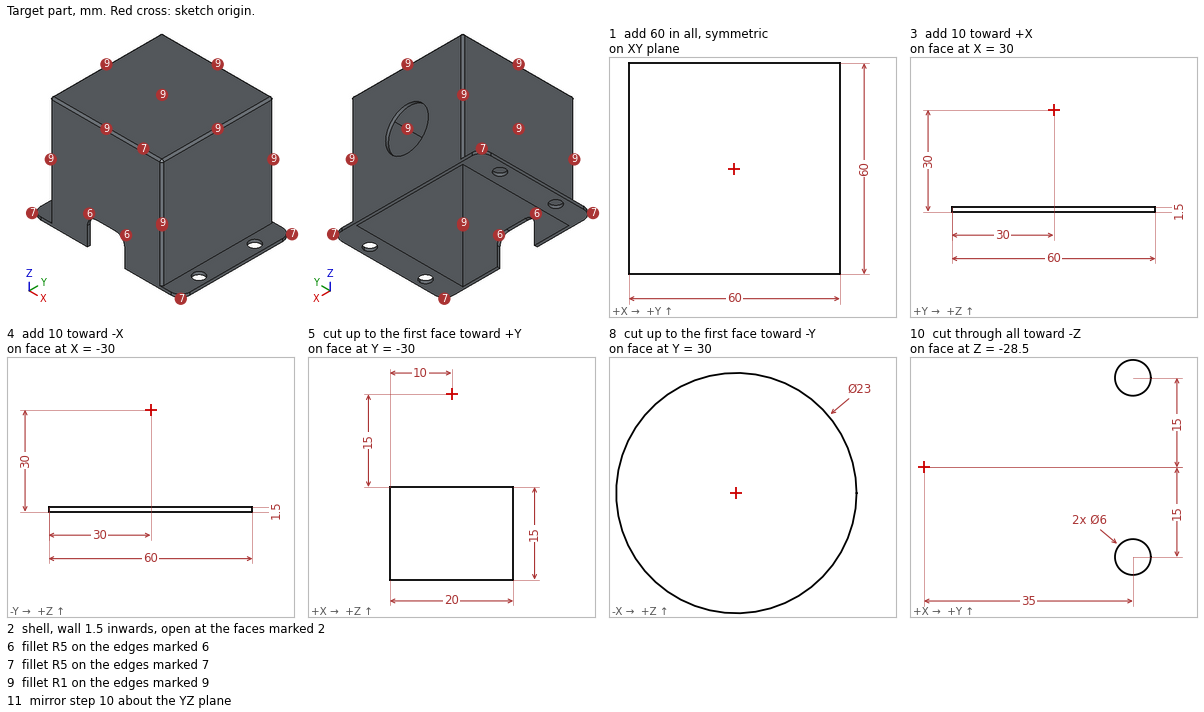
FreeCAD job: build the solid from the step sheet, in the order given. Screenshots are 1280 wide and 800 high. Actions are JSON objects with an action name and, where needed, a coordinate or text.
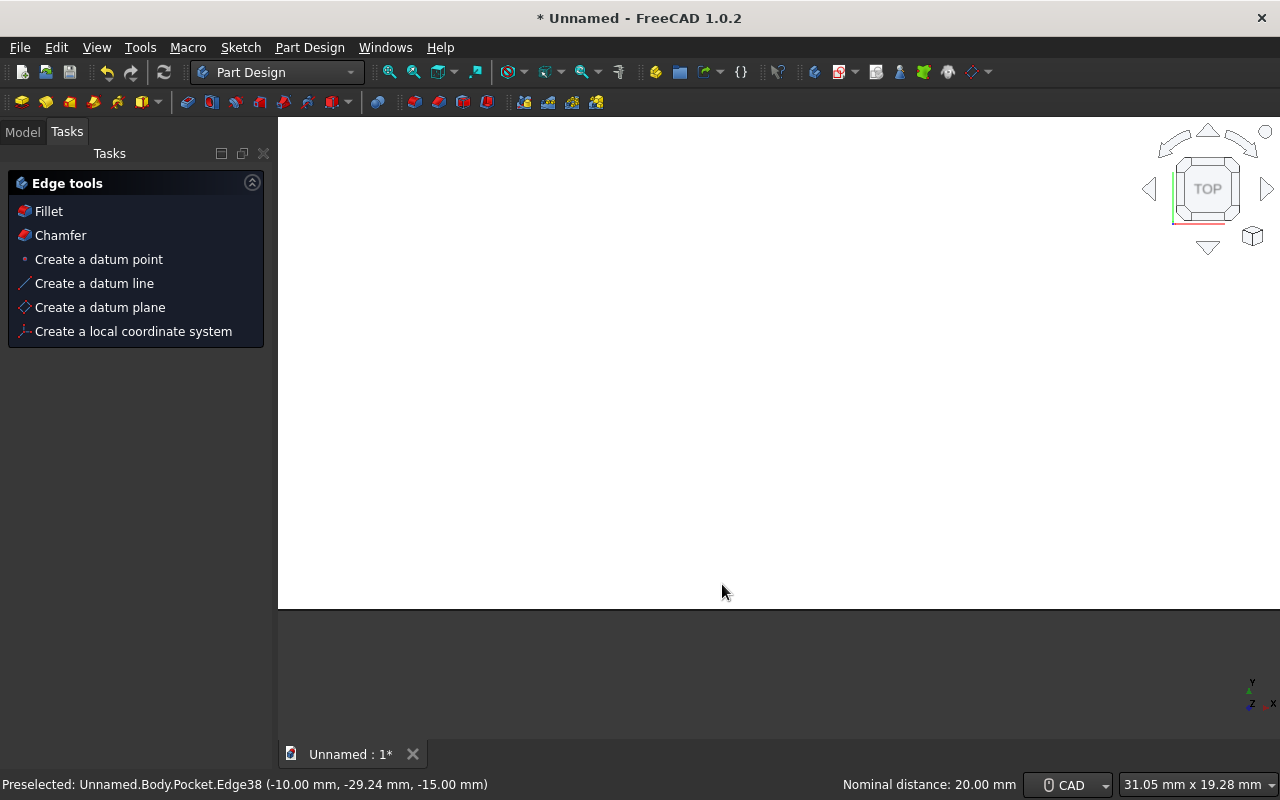
{"action": "left_click", "coordinate": [416, 102]}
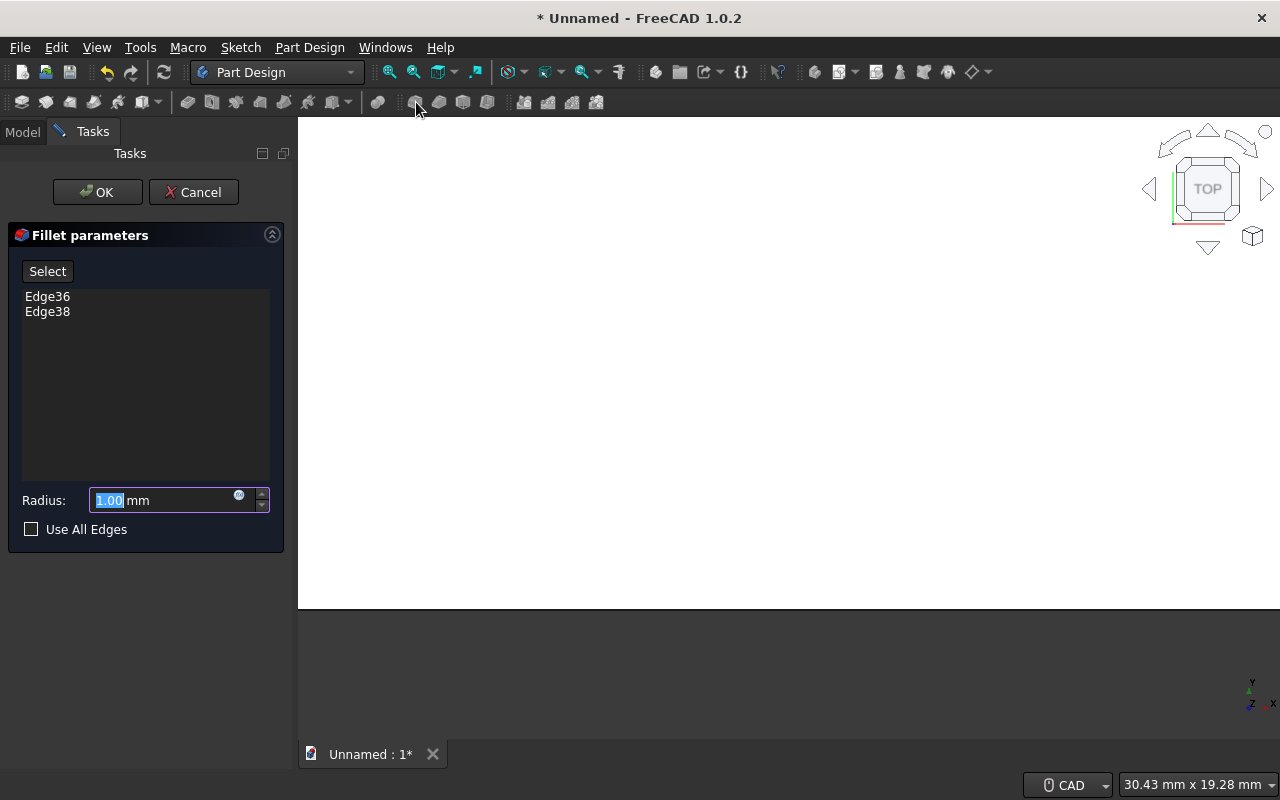
{"action": "type", "text": "5"}
{"action": "key", "text": "Tab"}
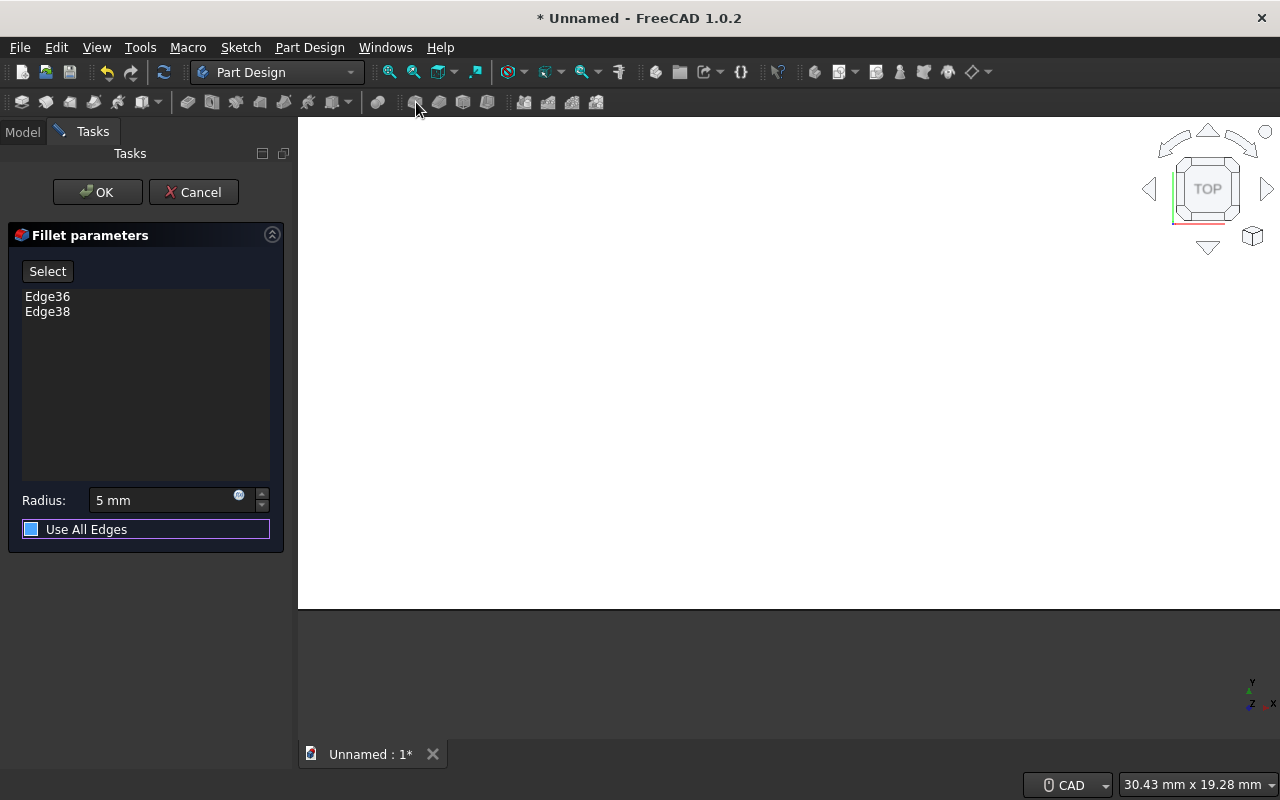
{"action": "left_click", "coordinate": [98, 192]}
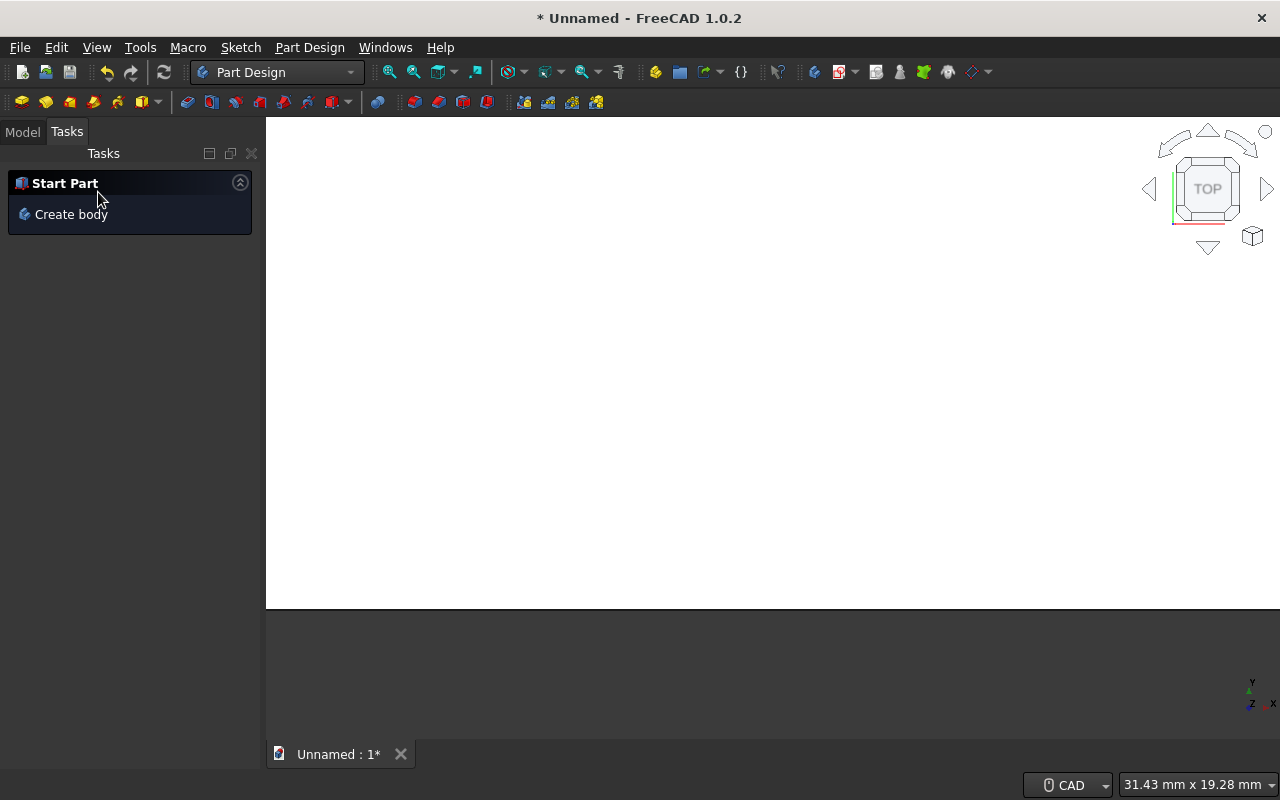
{"action": "key", "text": "v f"}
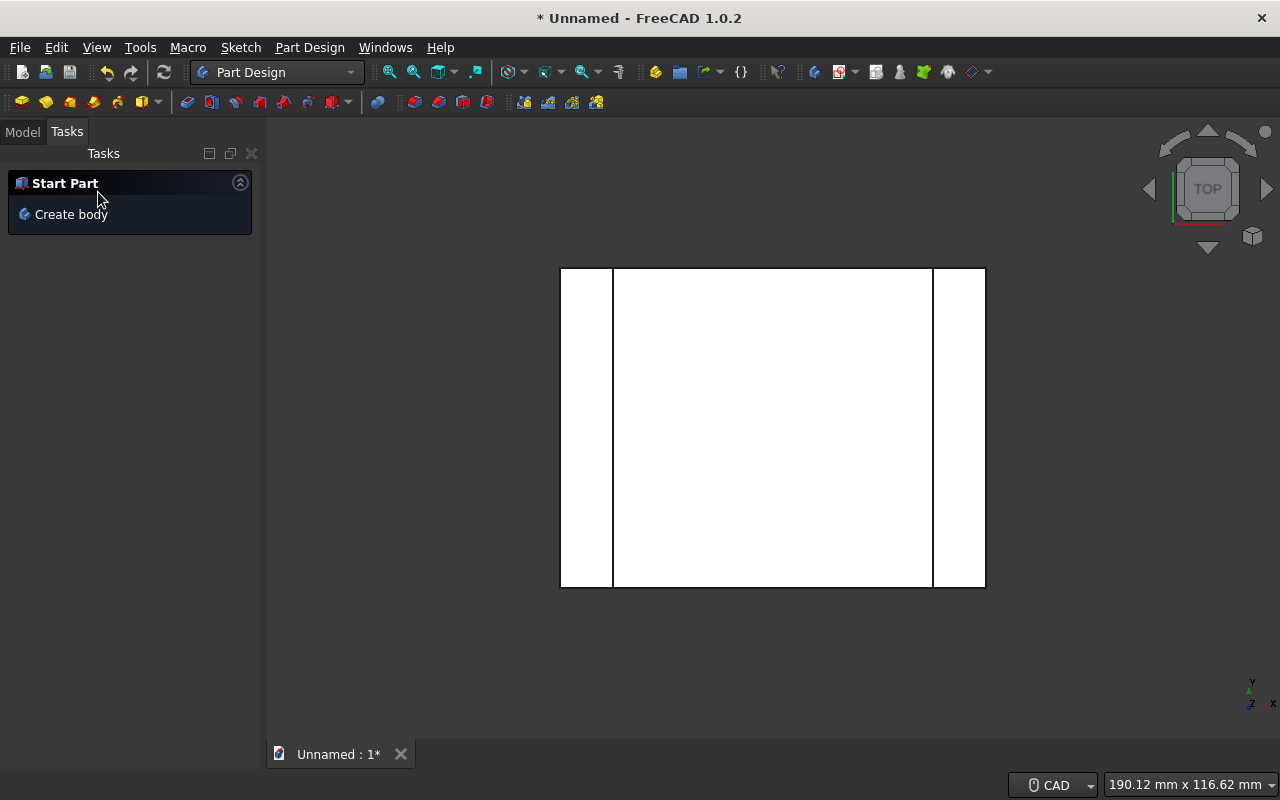
{"action": "scroll", "coordinate": [986, 267], "scroll_direction": "up", "scroll_amount": 9}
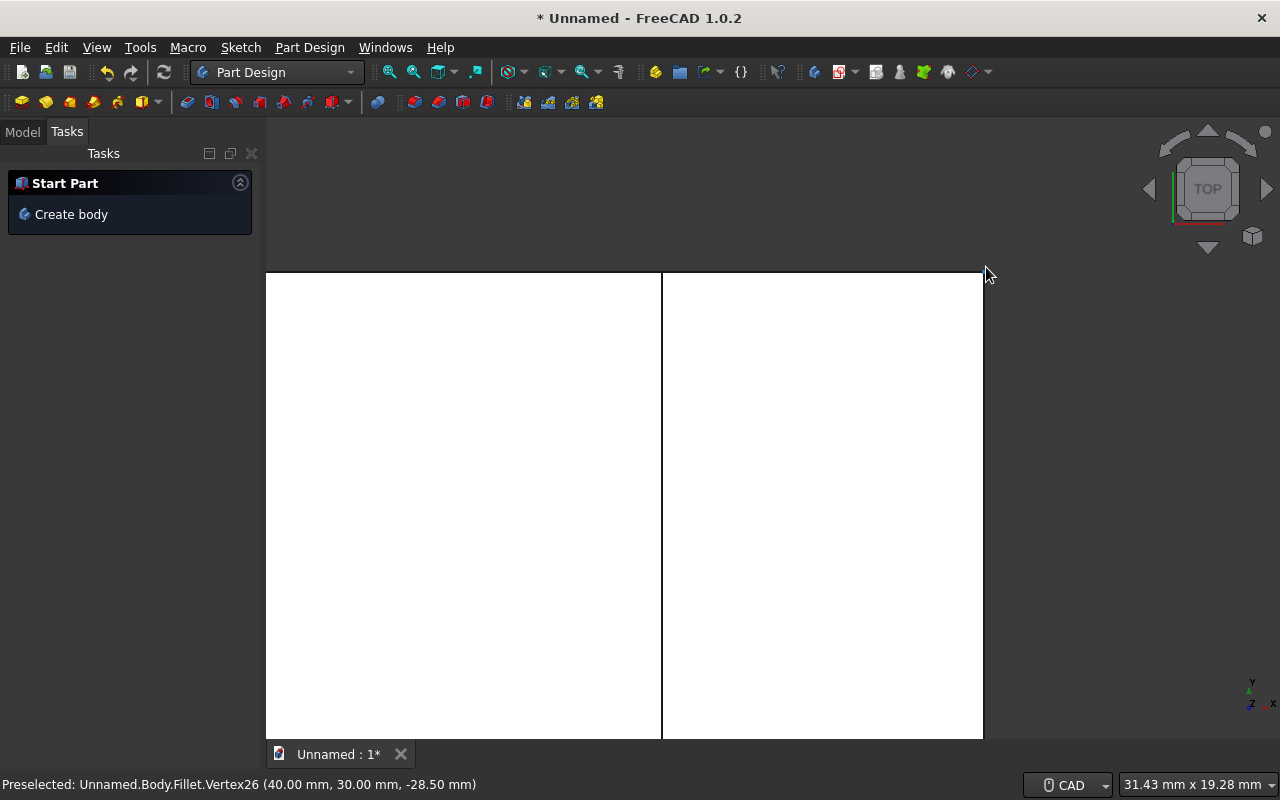
{"action": "key", "text": "v f"}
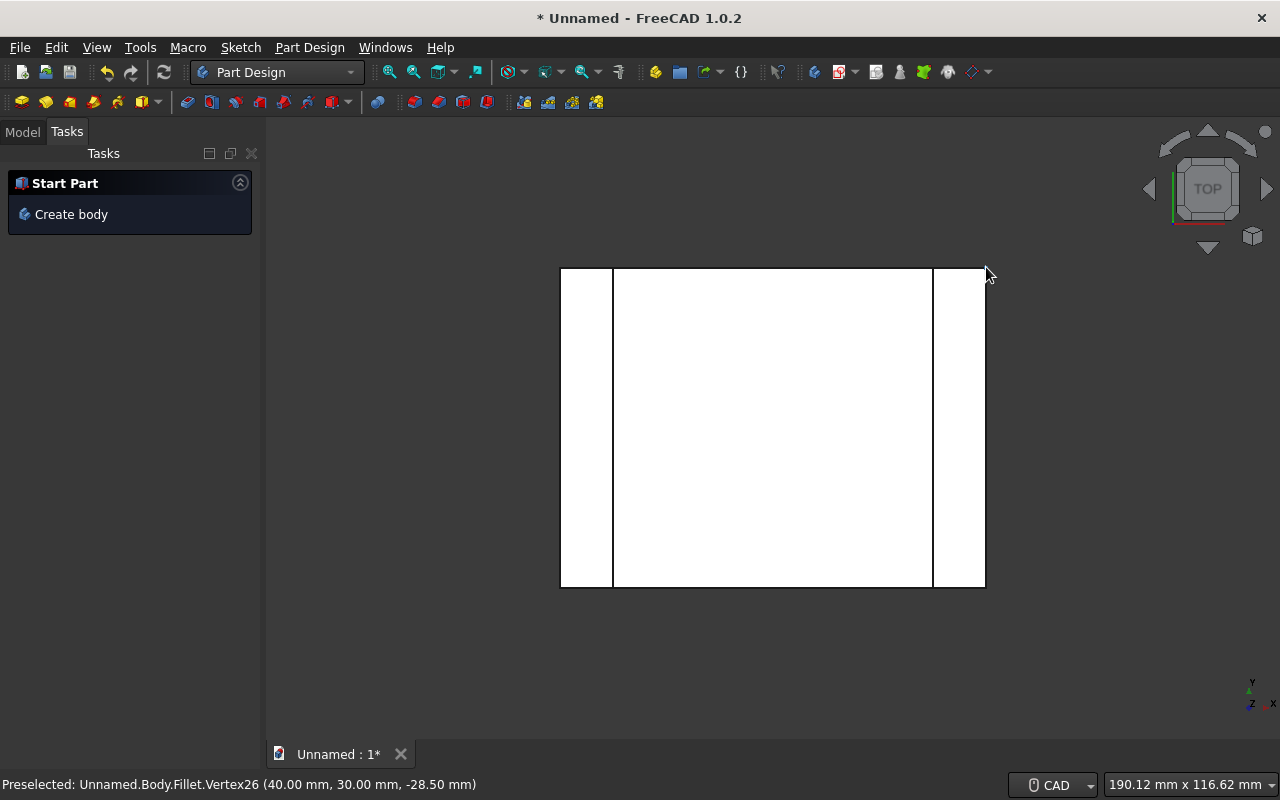
{"action": "key", "text": "0"}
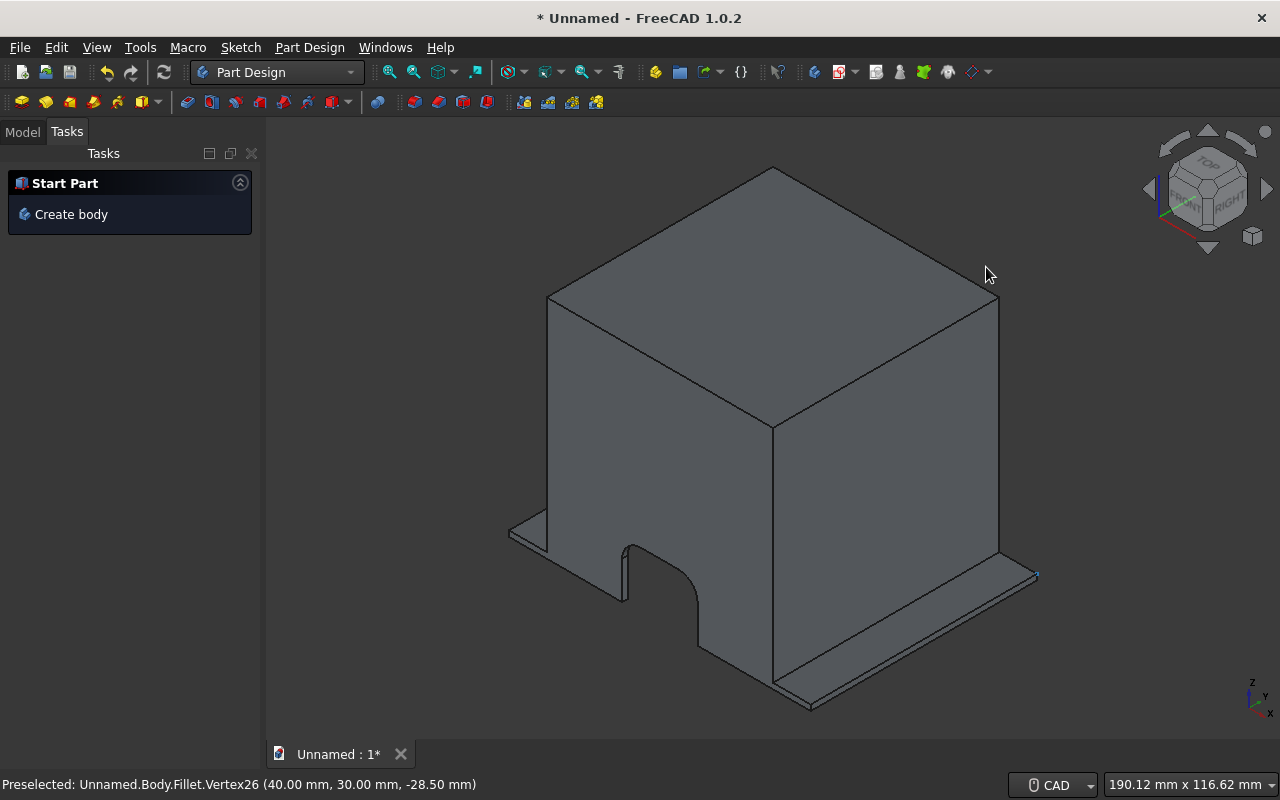
{"action": "scroll", "coordinate": [1037, 576], "scroll_direction": "up", "scroll_amount": 9}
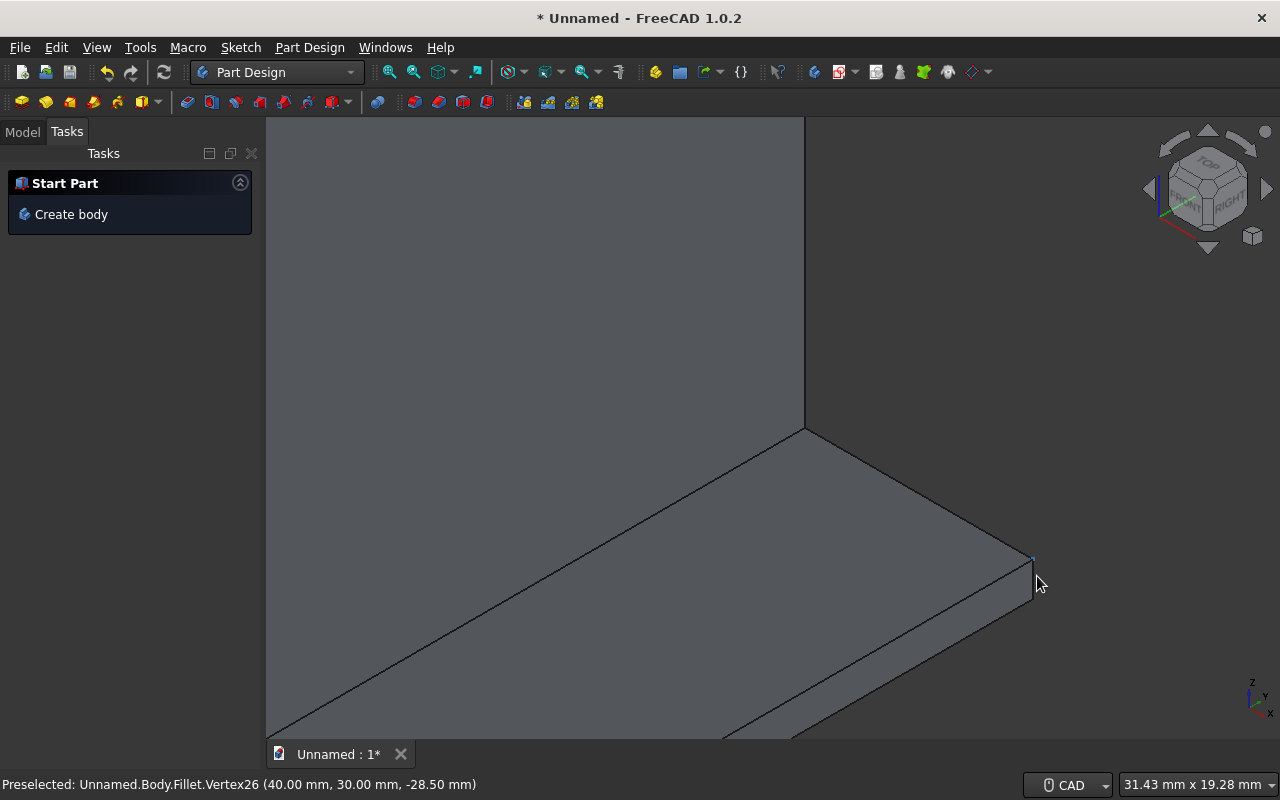
{"action": "key", "text": "v f"}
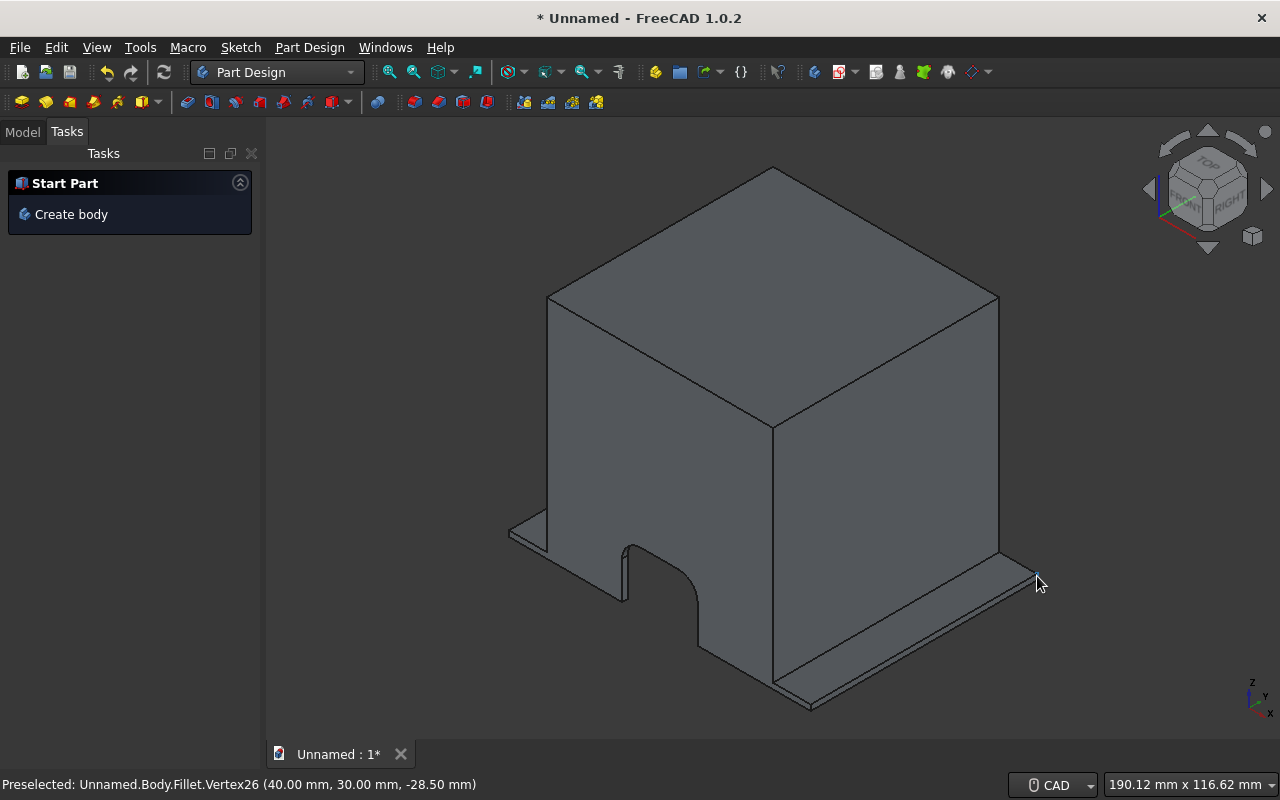
{"action": "key", "text": "2"}